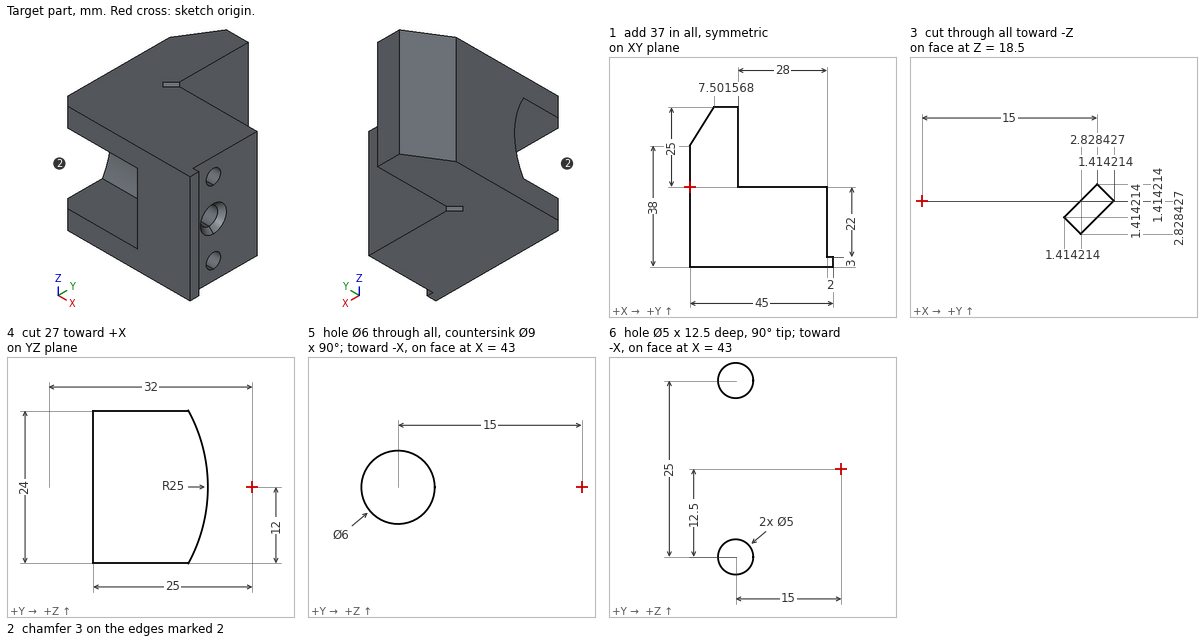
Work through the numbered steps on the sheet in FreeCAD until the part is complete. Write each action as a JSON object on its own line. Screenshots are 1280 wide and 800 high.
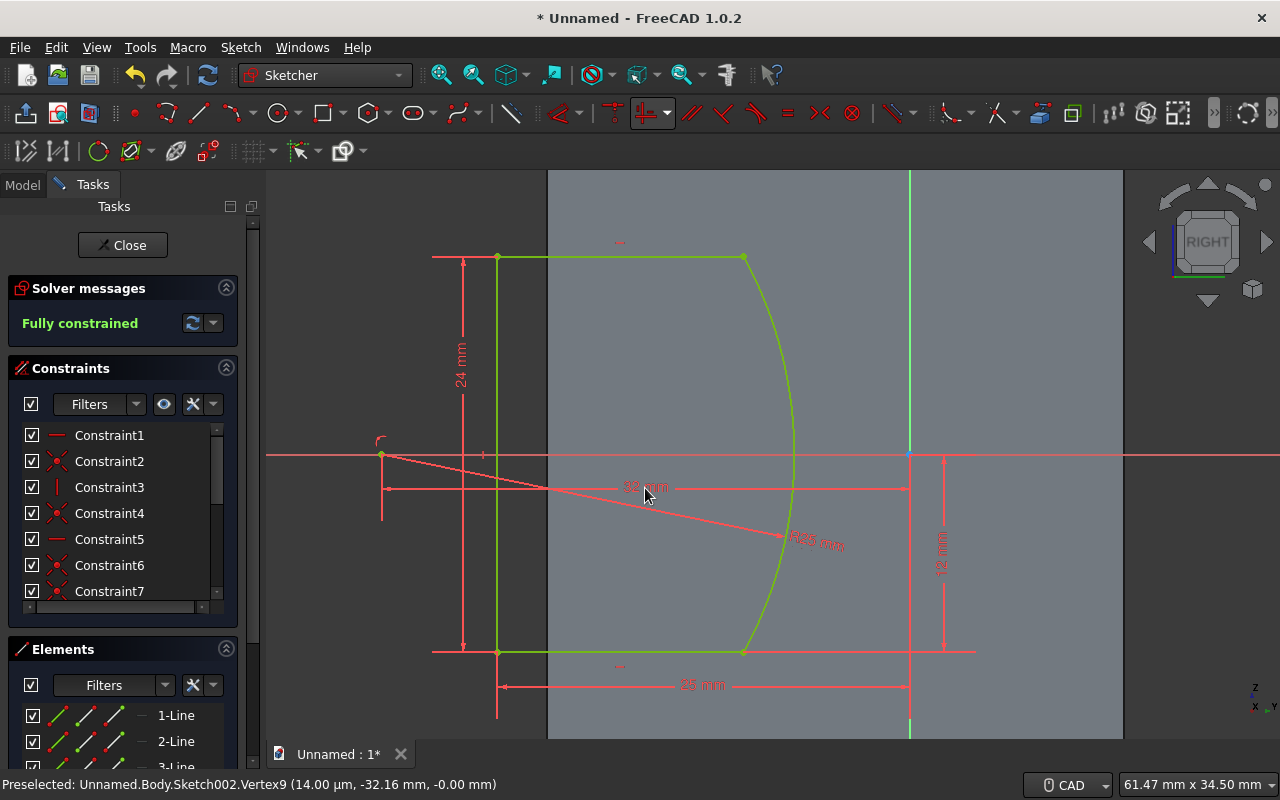
{"action": "left_click", "coordinate": [123, 245]}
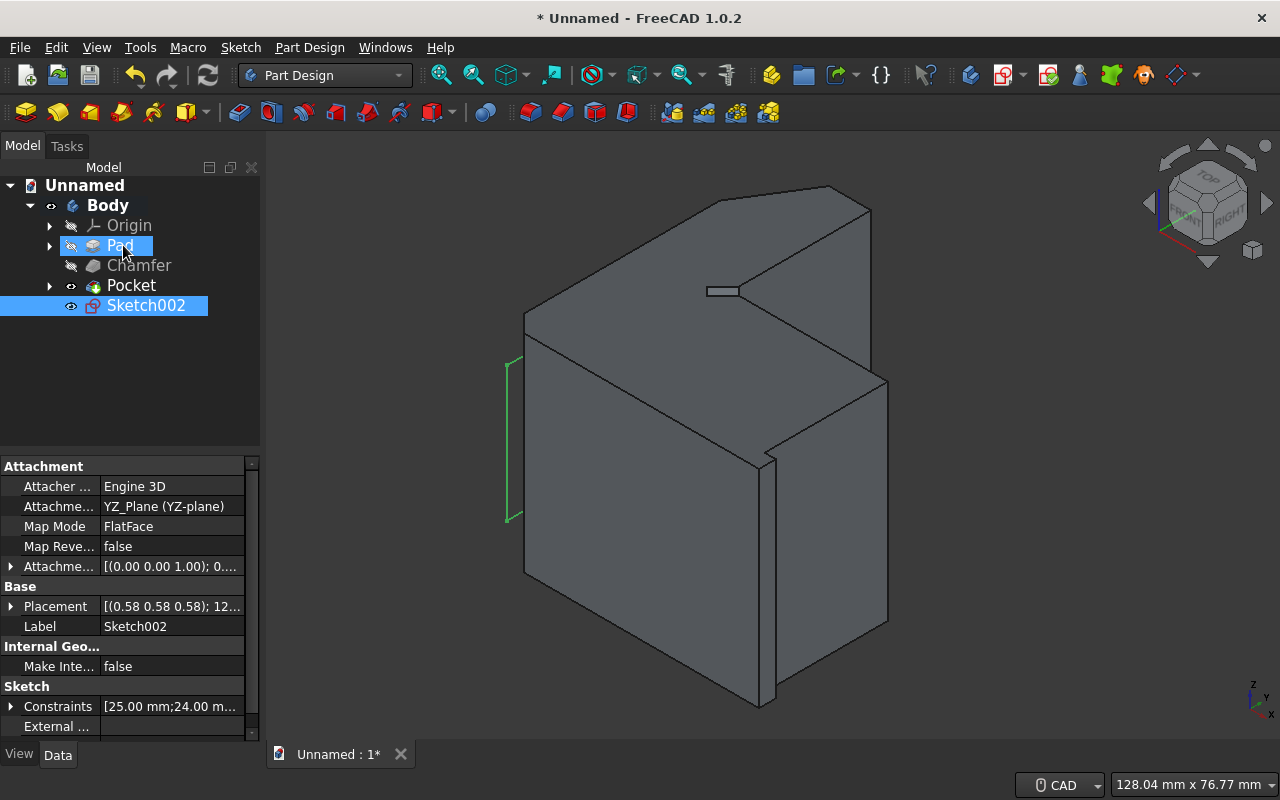
{"action": "left_click", "coordinate": [240, 112]}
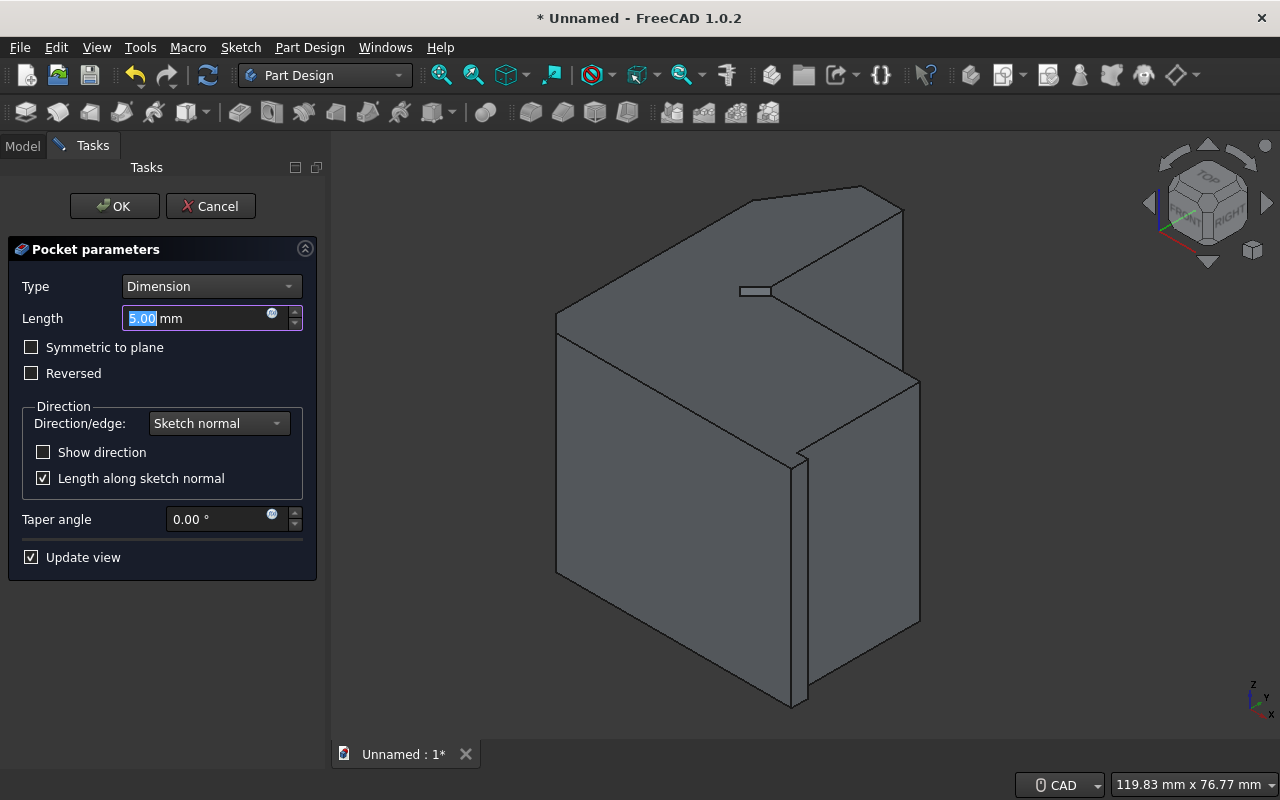
{"action": "type", "text": "27"}
{"action": "key", "text": "Tab"}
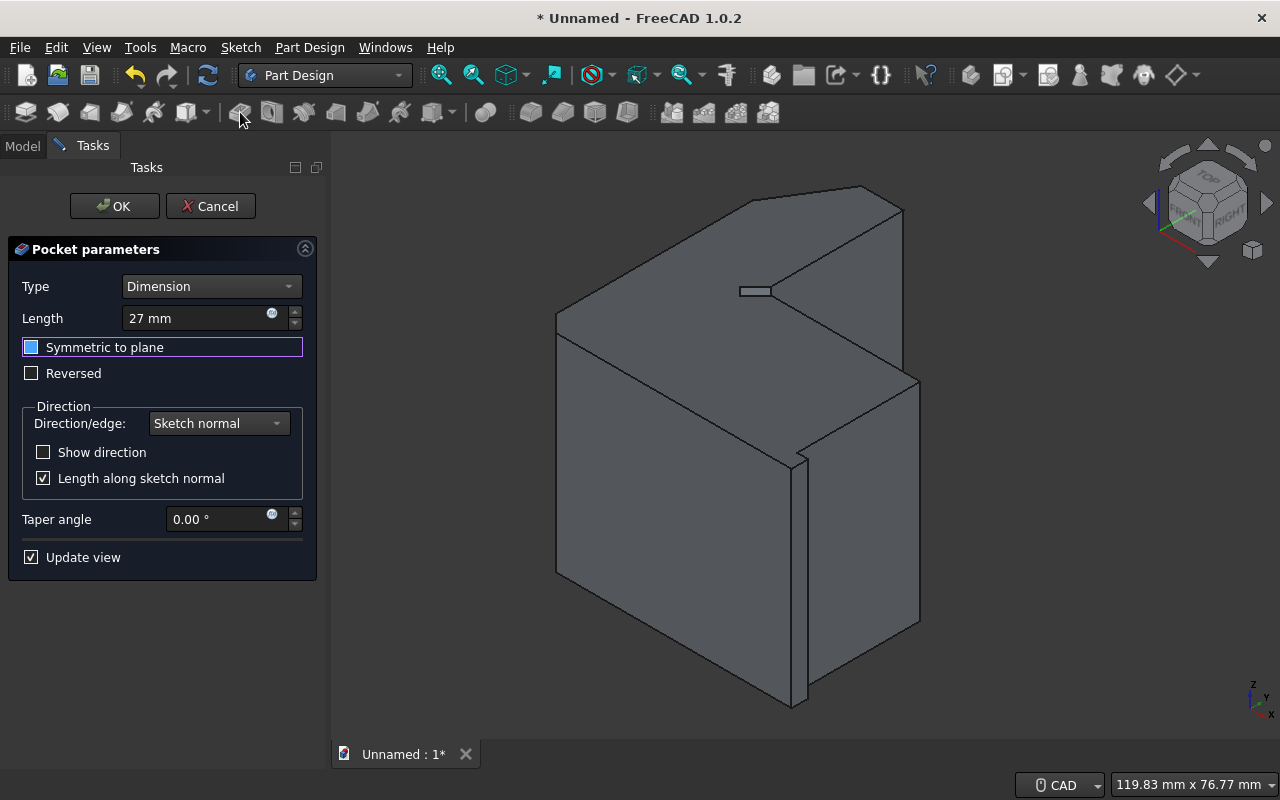
{"action": "left_click", "coordinate": [30, 373]}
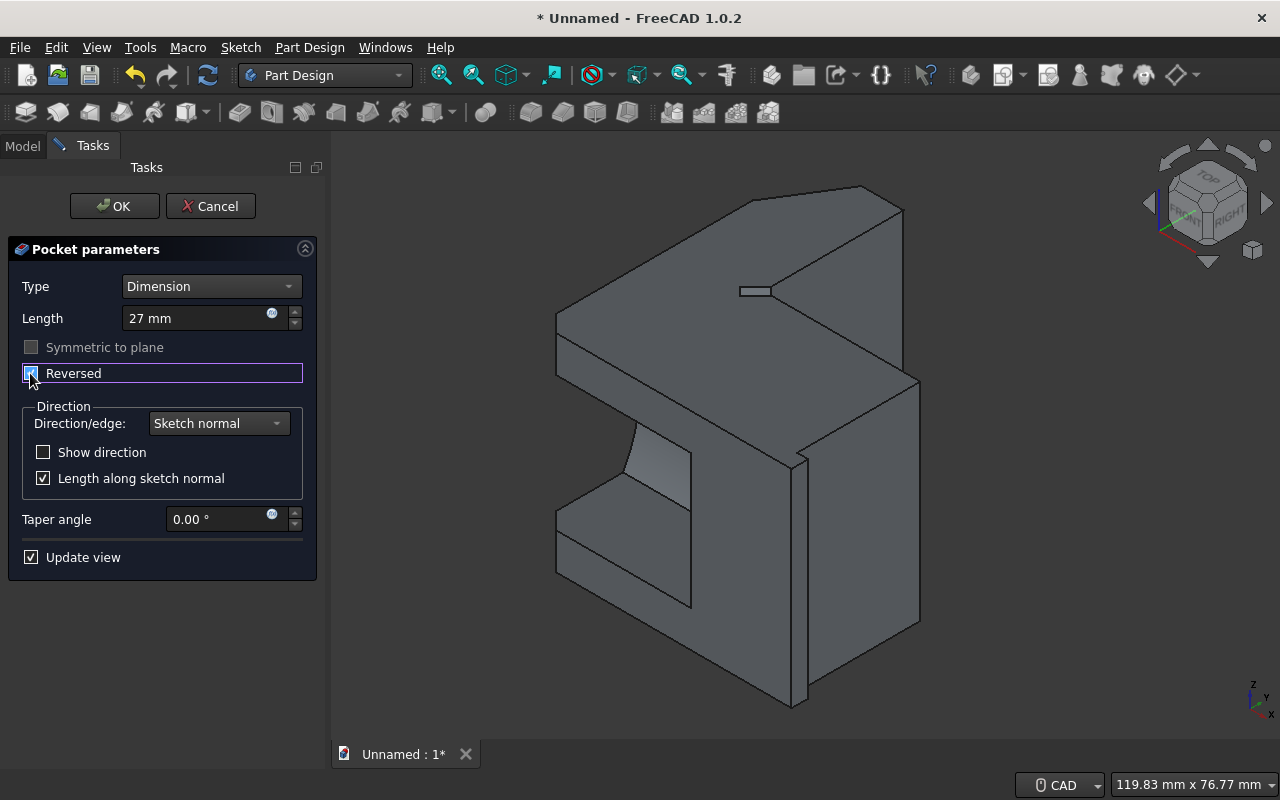
{"action": "left_click", "coordinate": [115, 206]}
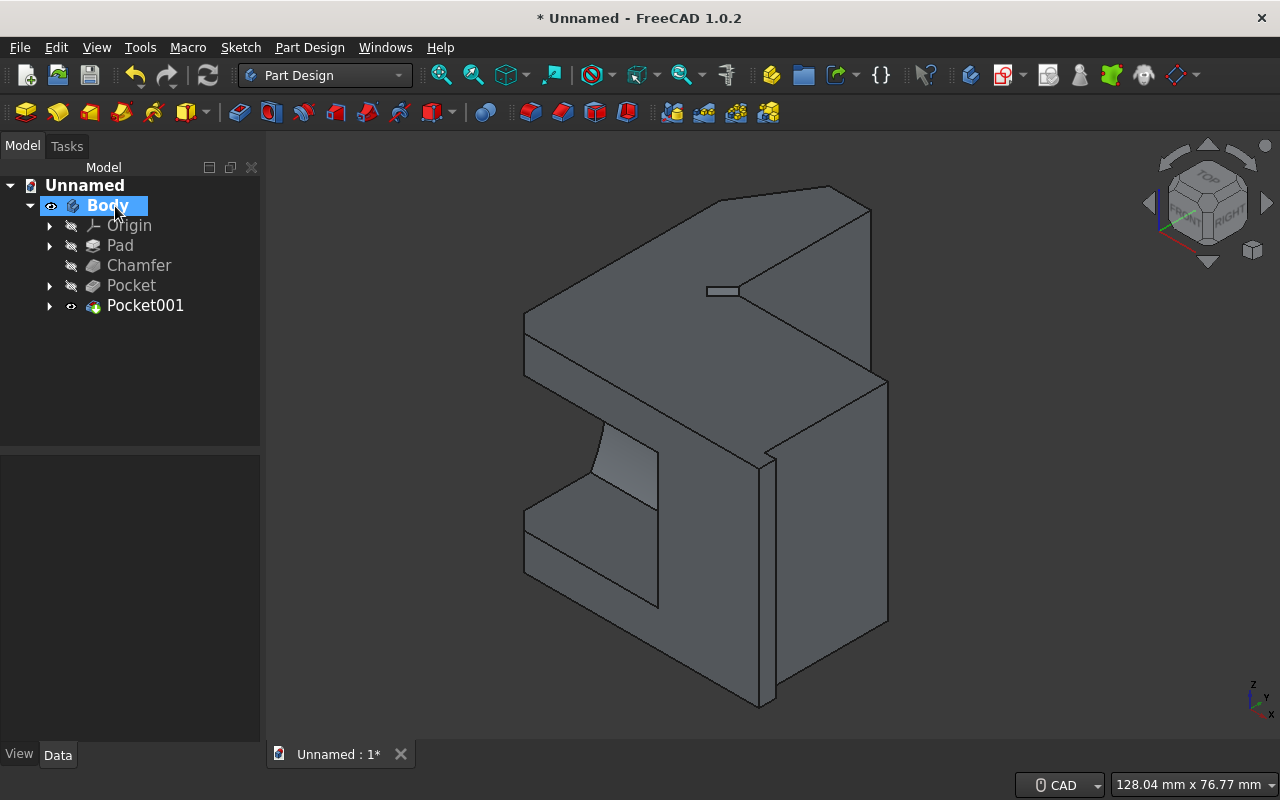
{"action": "left_click", "coordinate": [826, 502]}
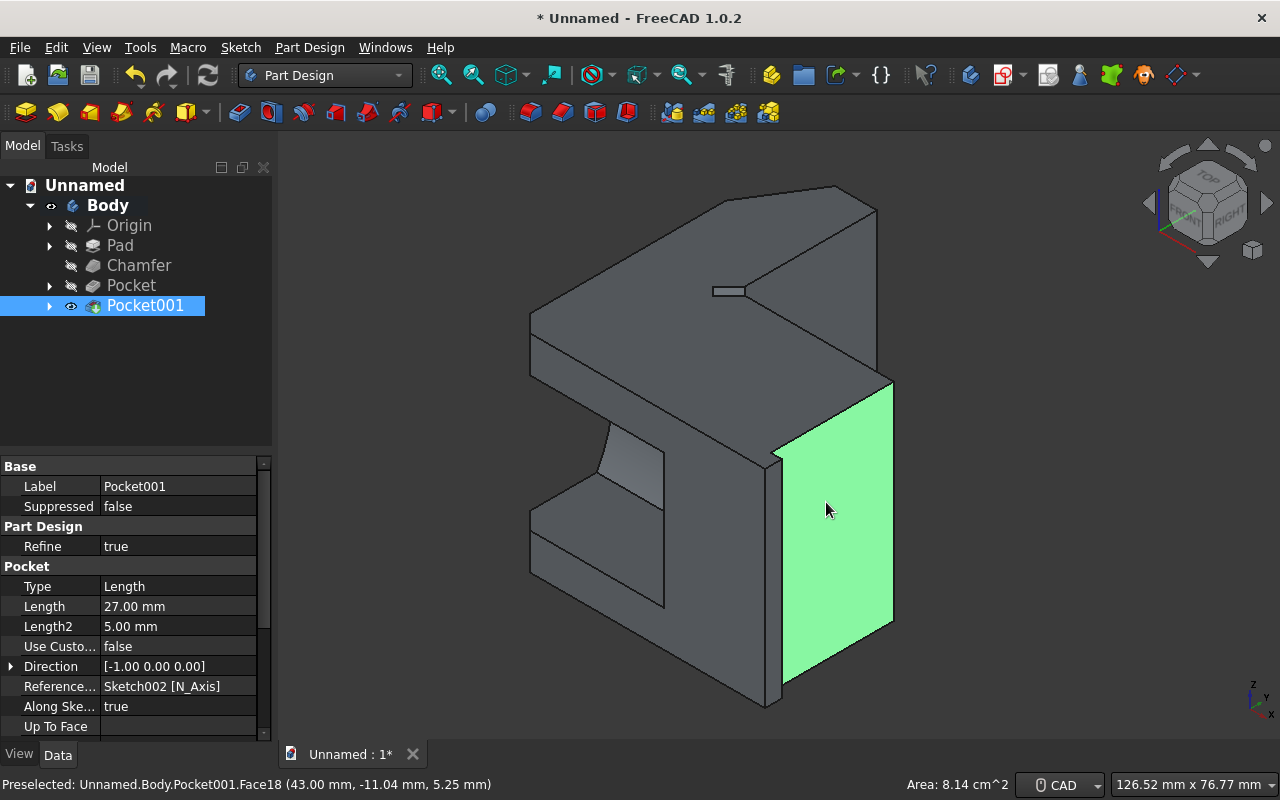
{"action": "left_click", "coordinate": [1004, 76]}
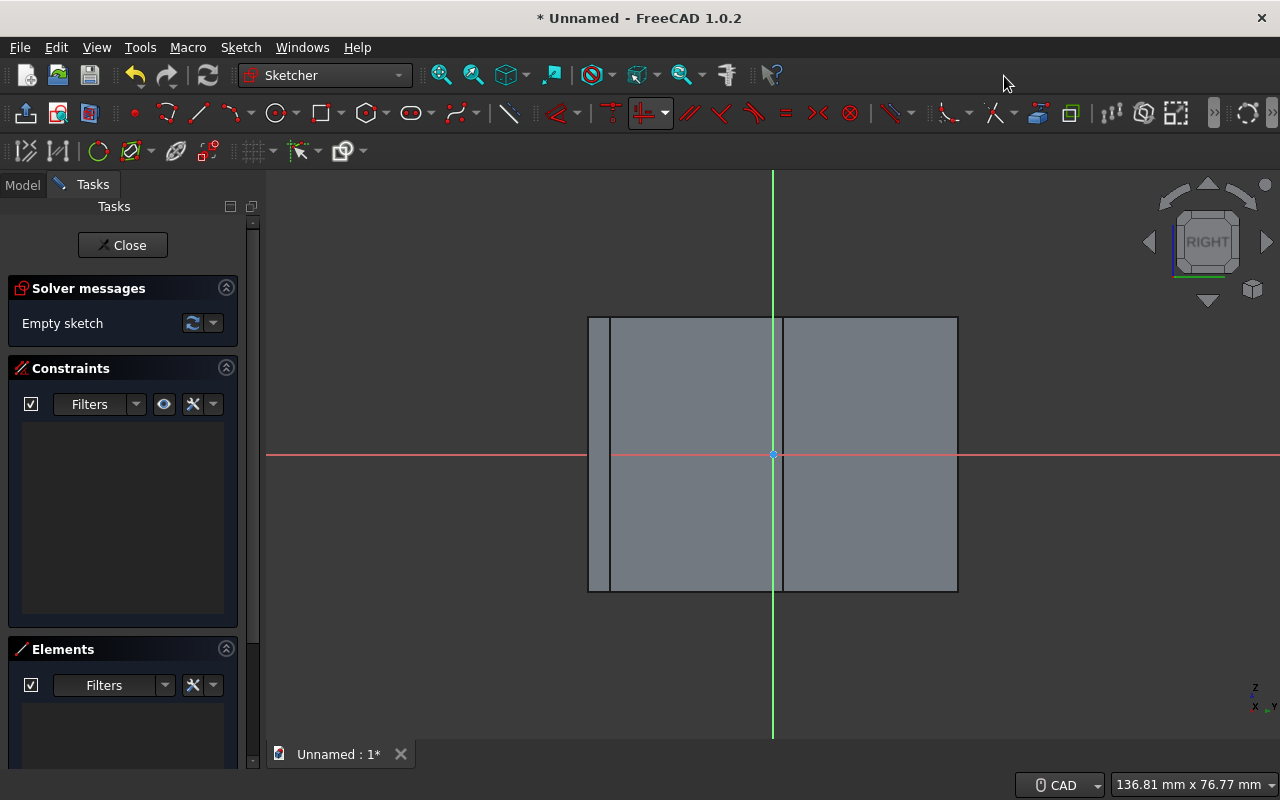
{"action": "scroll", "coordinate": [655, 454], "scroll_direction": "up", "scroll_amount": 10}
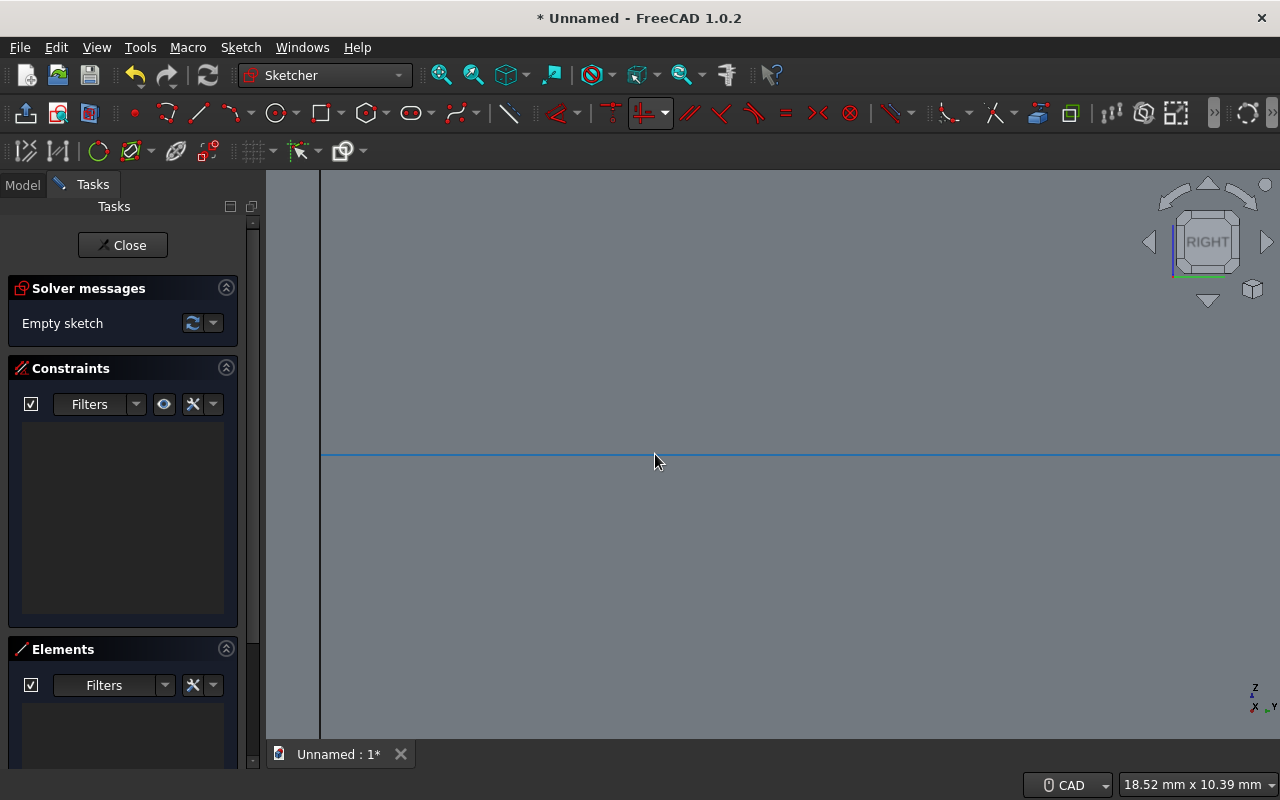
{"action": "left_click", "coordinate": [276, 114]}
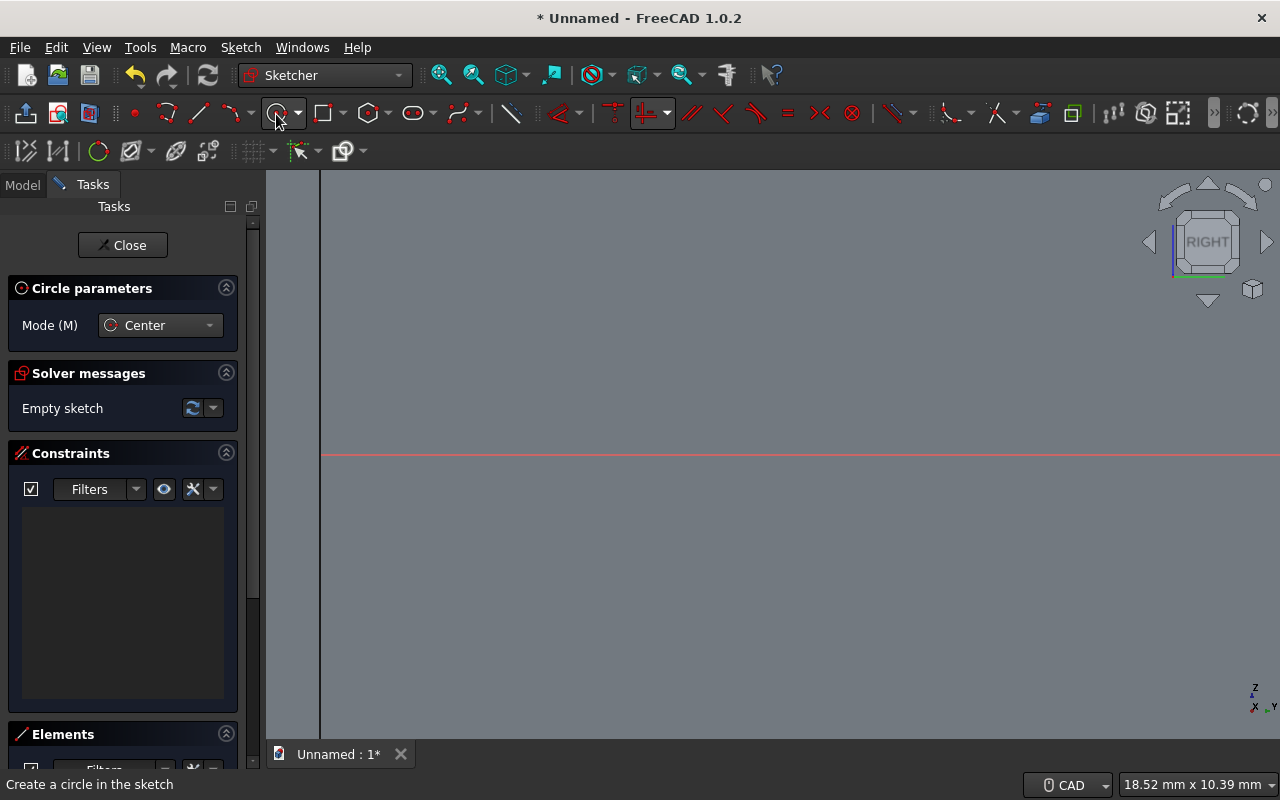
{"action": "left_click", "coordinate": [703, 454]}
{"action": "left_click", "coordinate": [819, 338]}
{"action": "key", "text": "Escape"}